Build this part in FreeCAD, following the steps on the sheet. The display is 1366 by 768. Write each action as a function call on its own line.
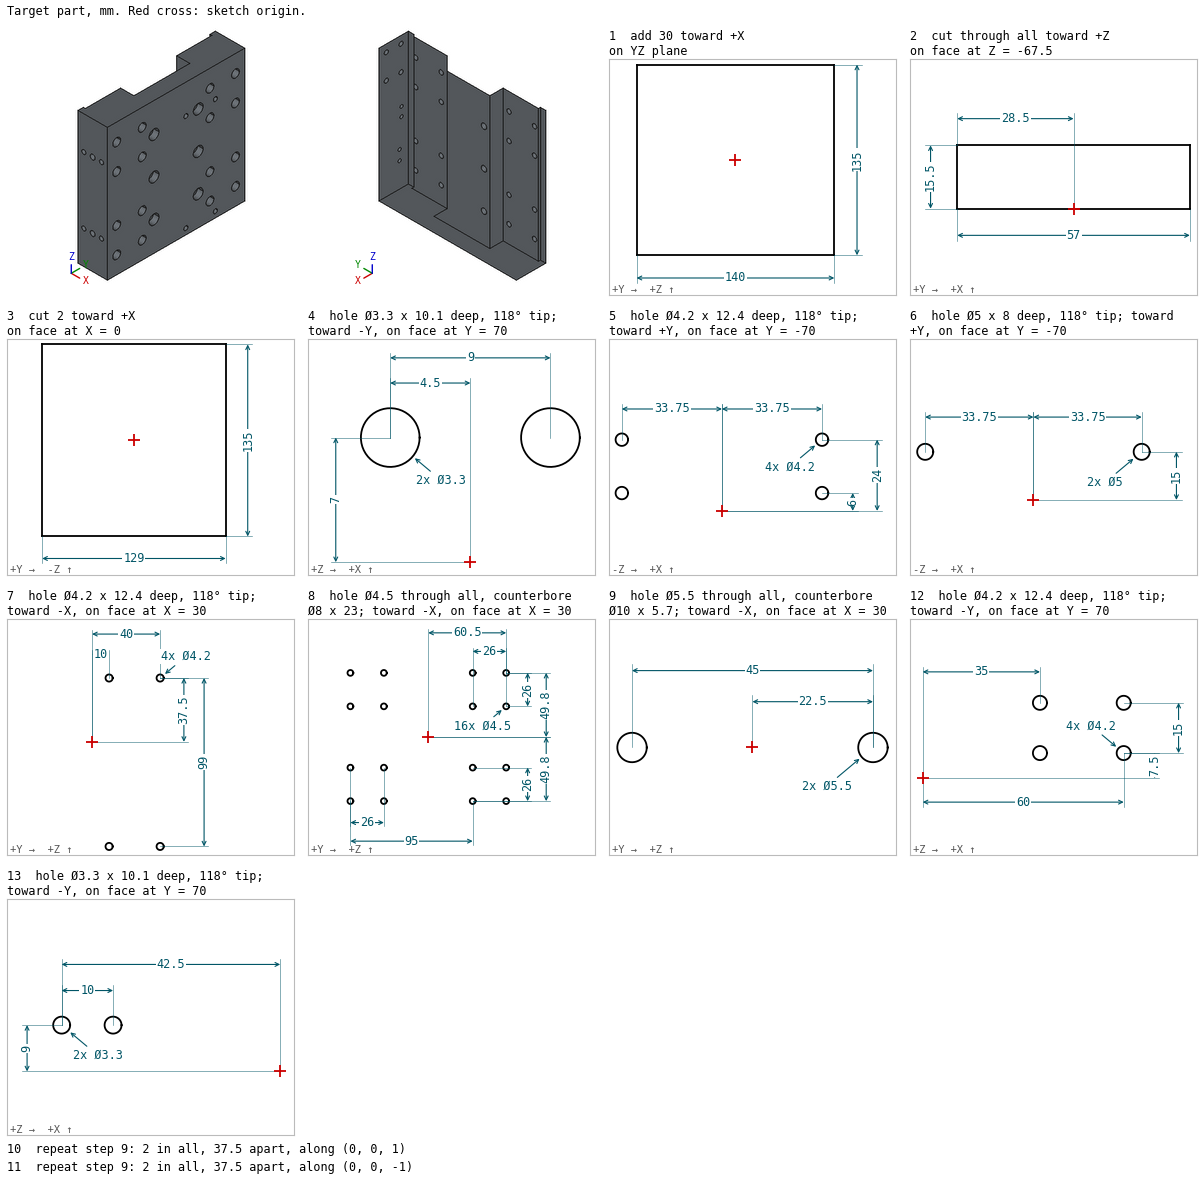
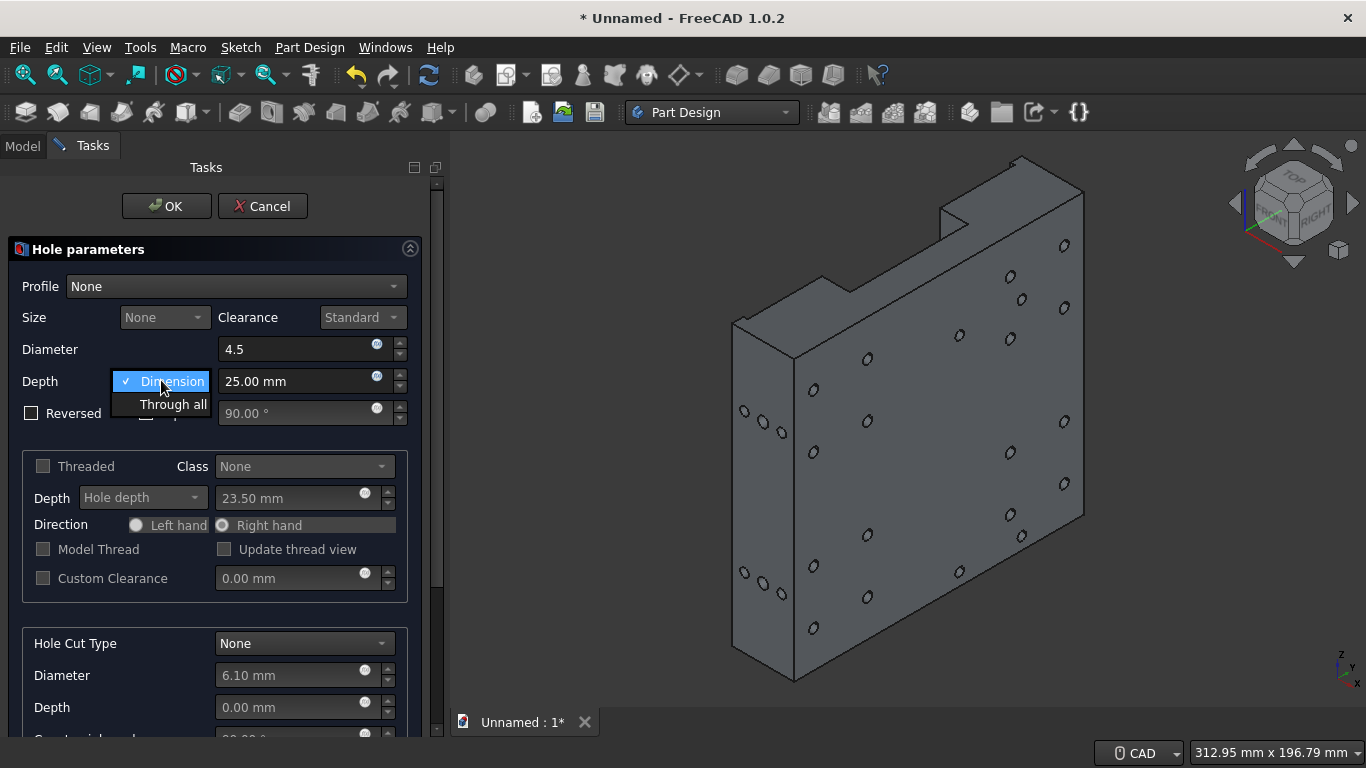
click(160, 404)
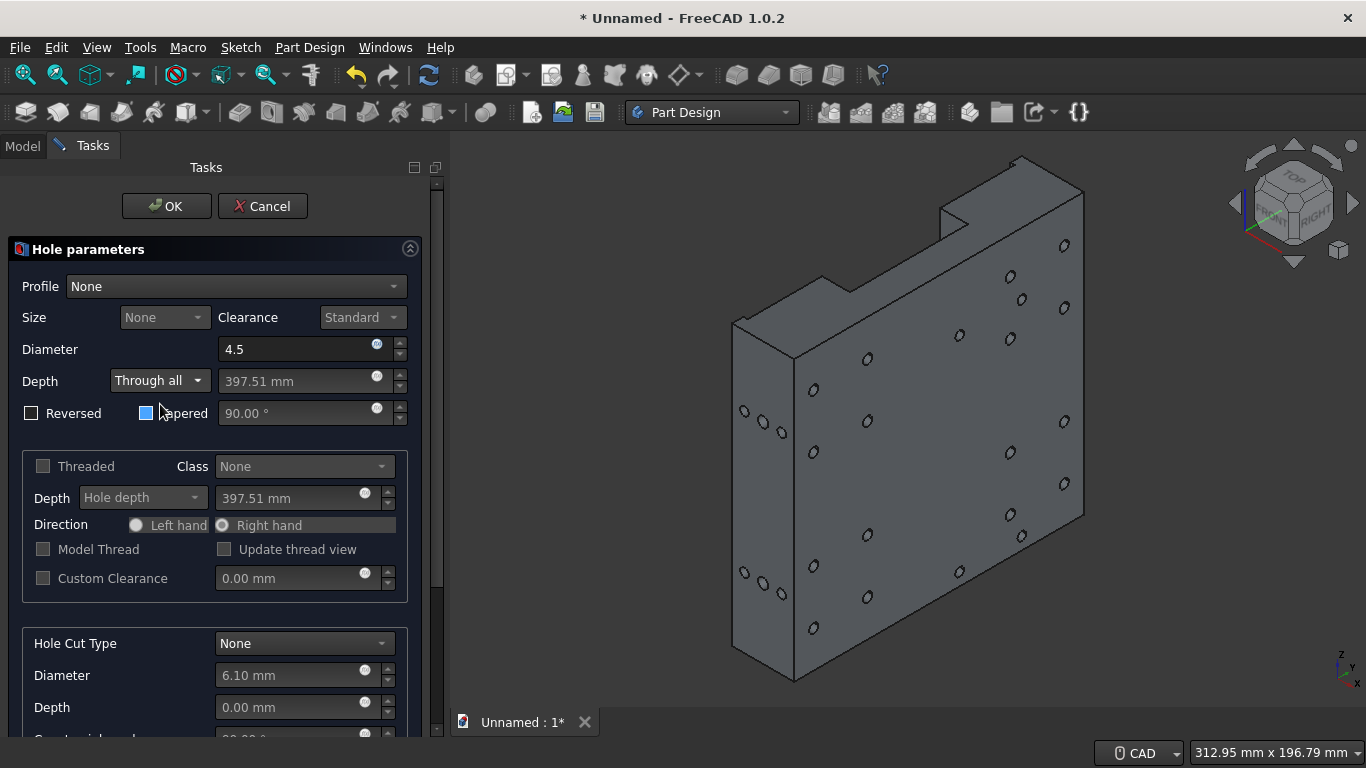
click(306, 644)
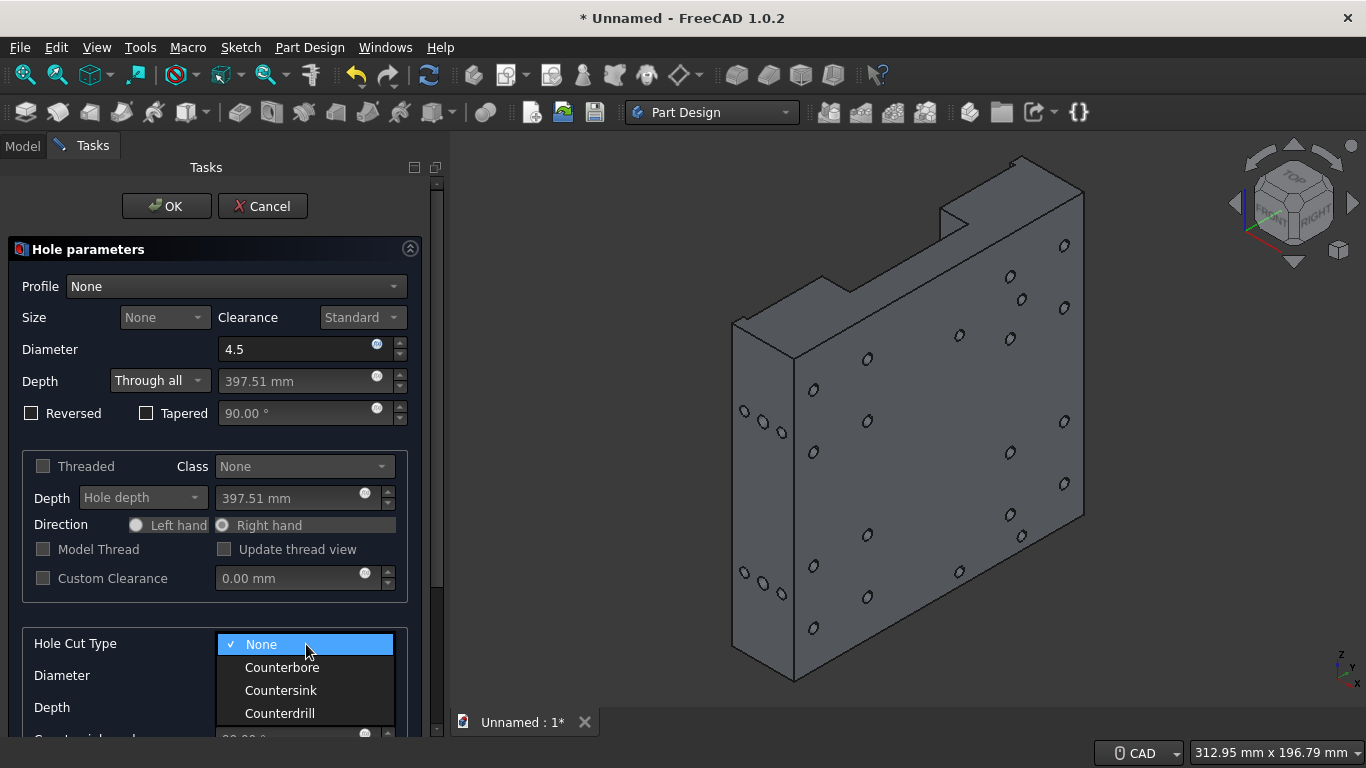
click(304, 668)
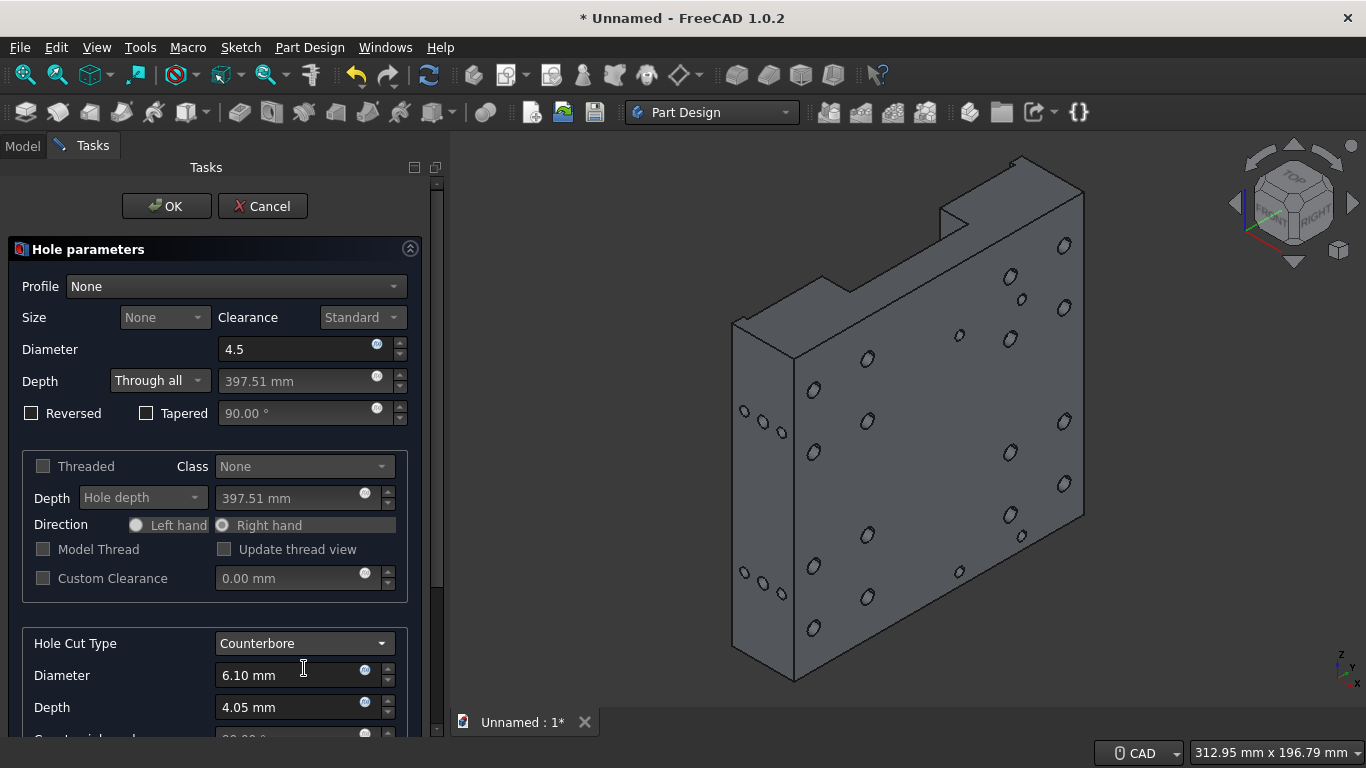
triple_click(298, 675)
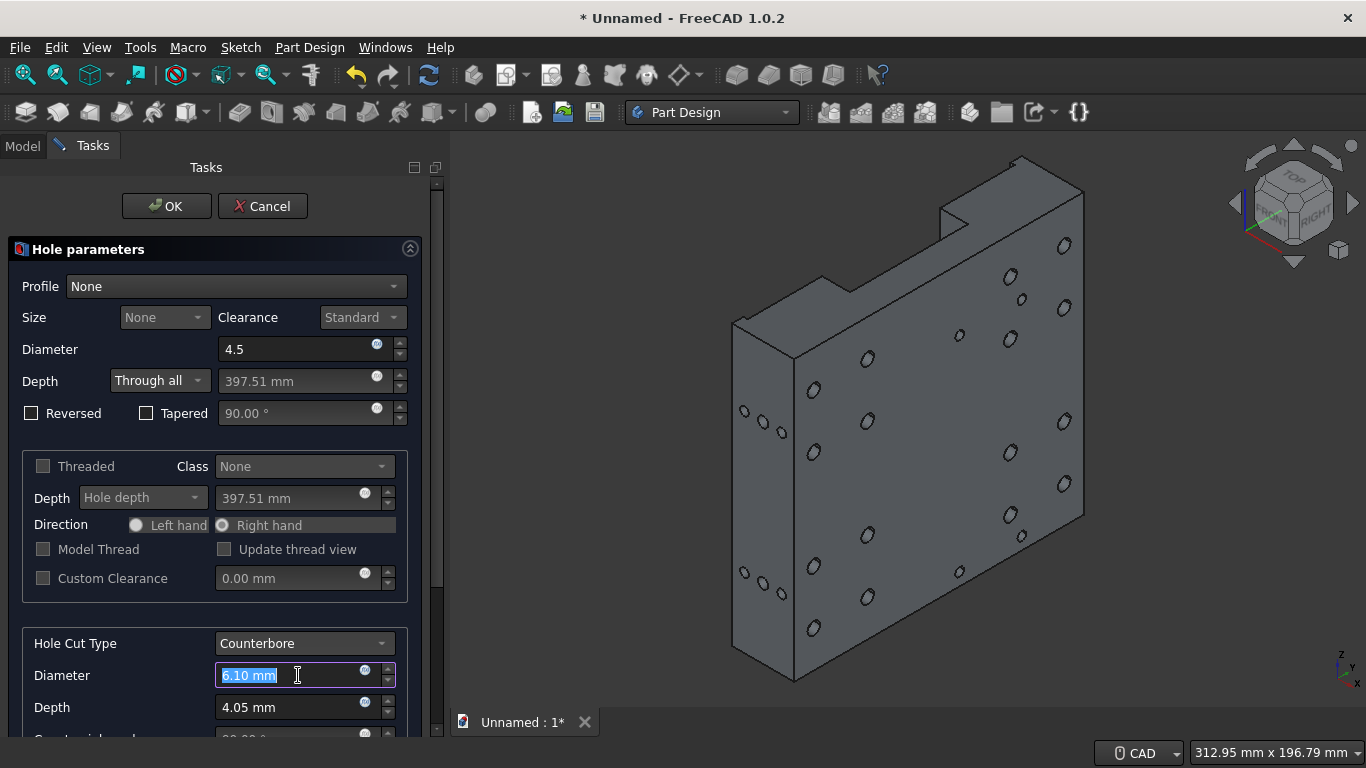
text(8)
key(Tab)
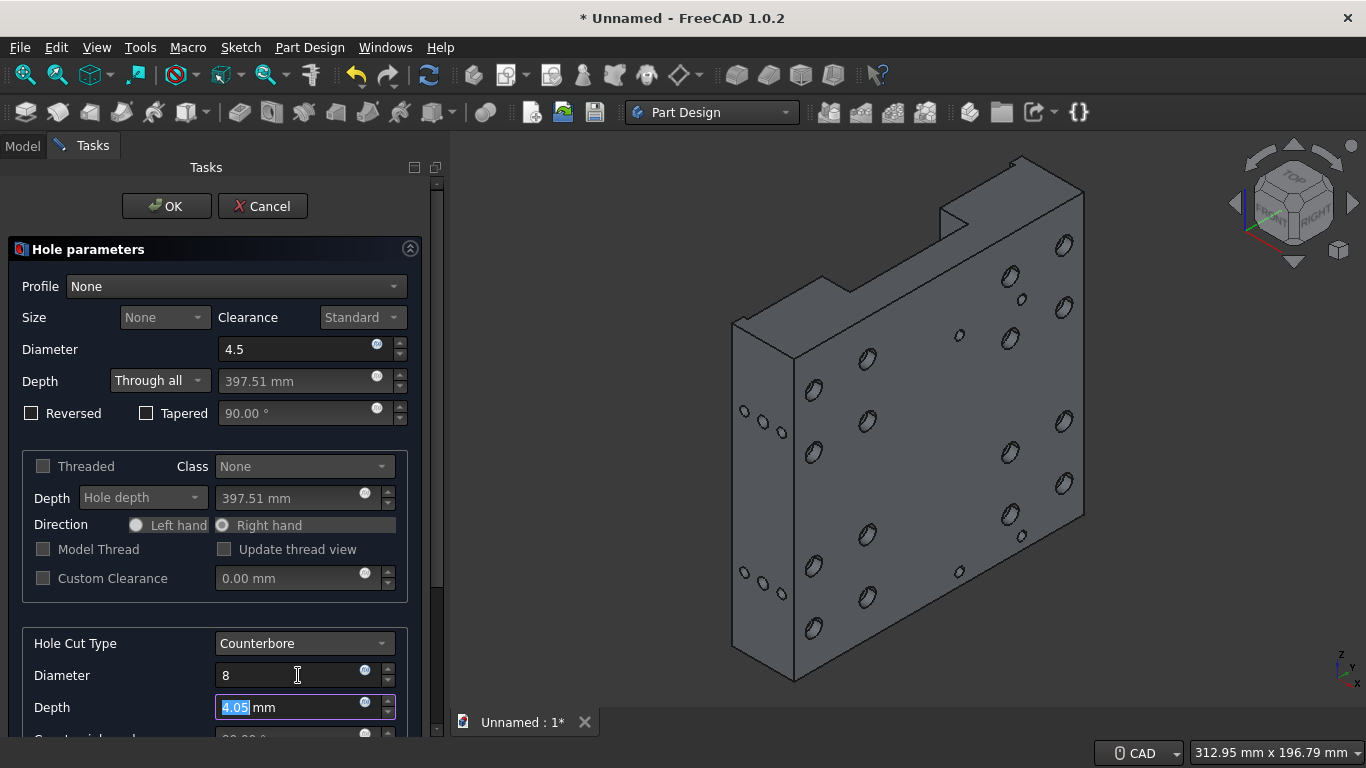
text(23)
key(Tab)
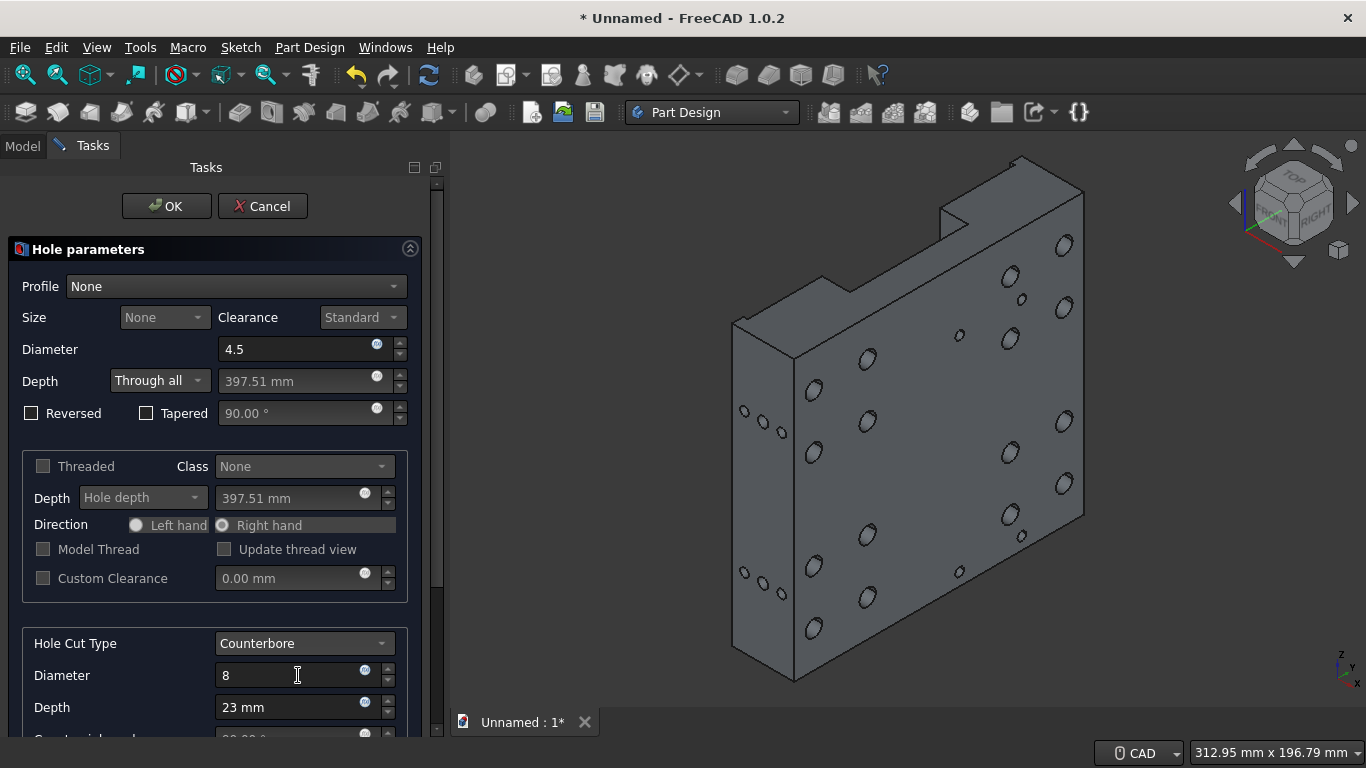
click(167, 206)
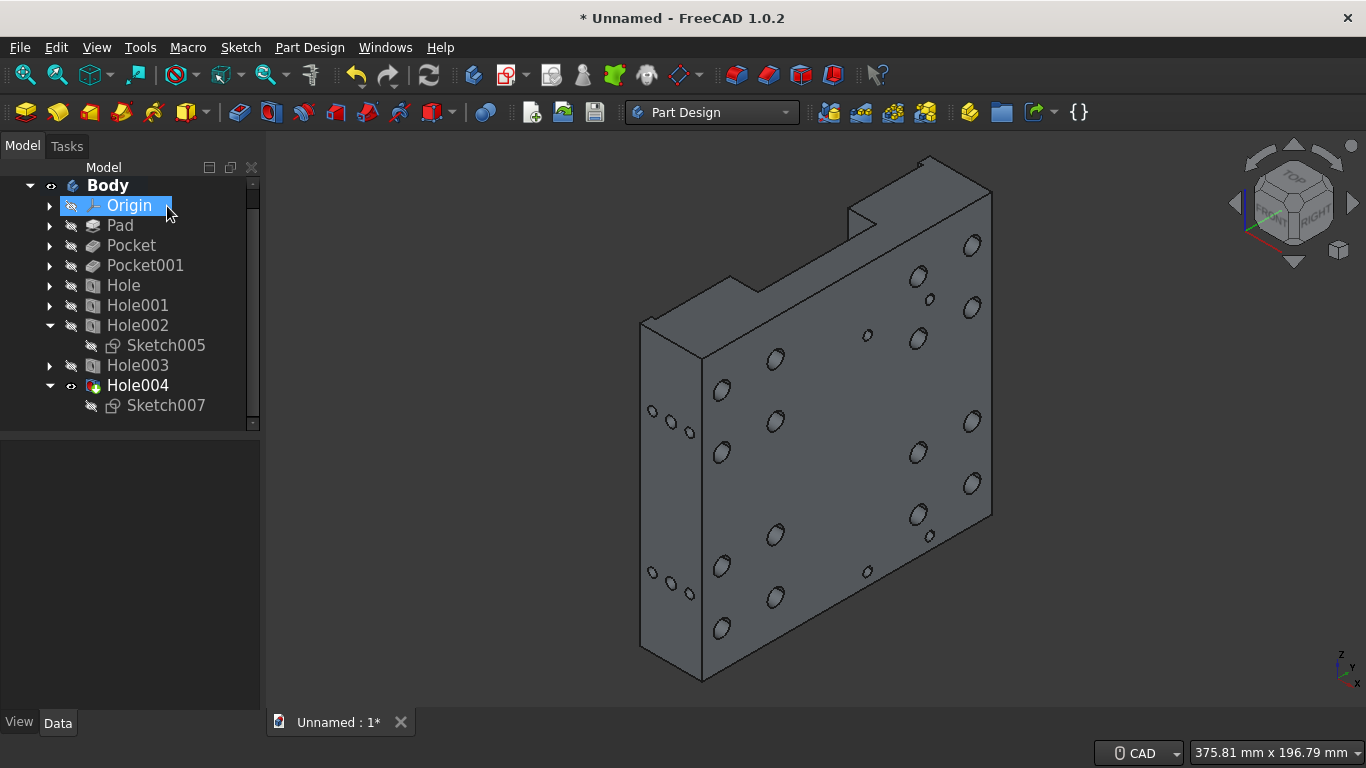
click(847, 436)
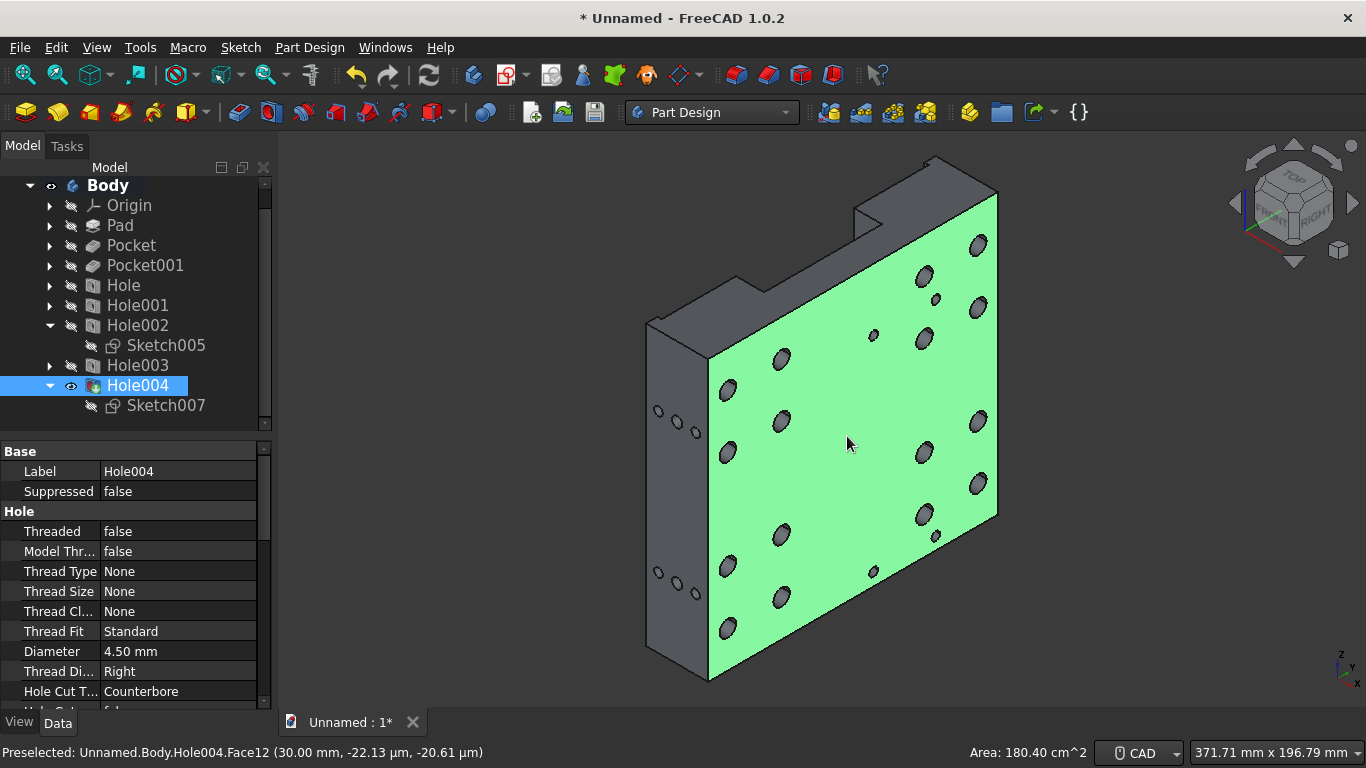
click(506, 76)